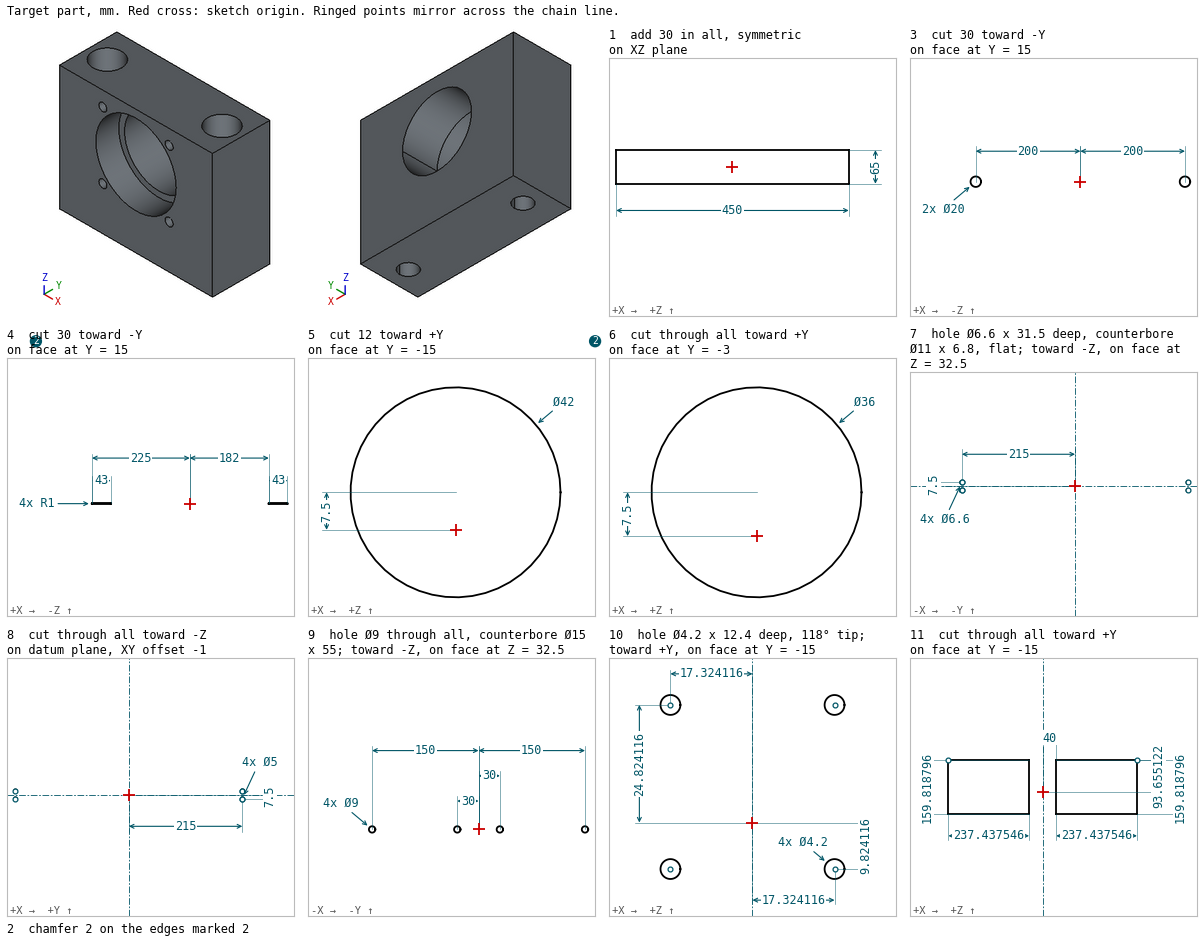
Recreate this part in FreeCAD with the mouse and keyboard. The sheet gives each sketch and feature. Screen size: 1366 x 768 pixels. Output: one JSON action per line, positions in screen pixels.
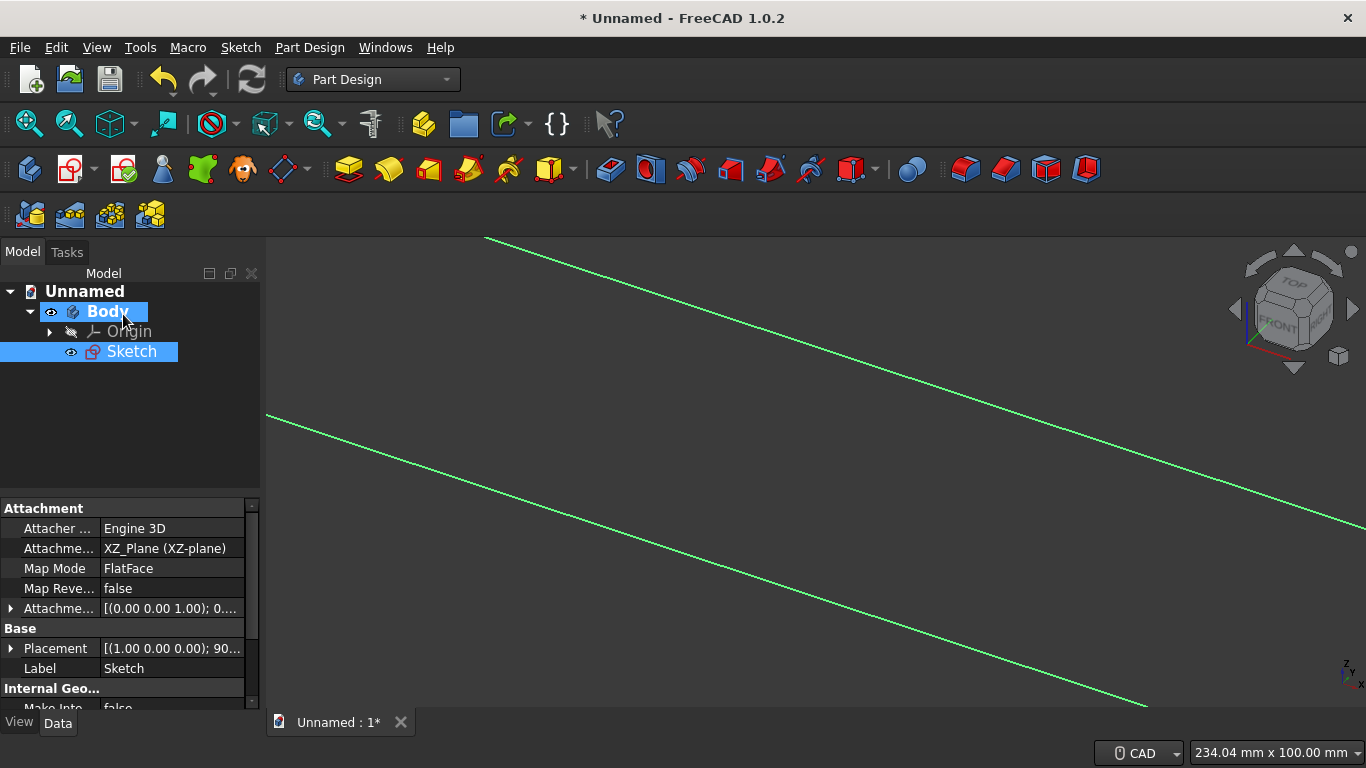
{"action": "left_click", "coordinate": [350, 170]}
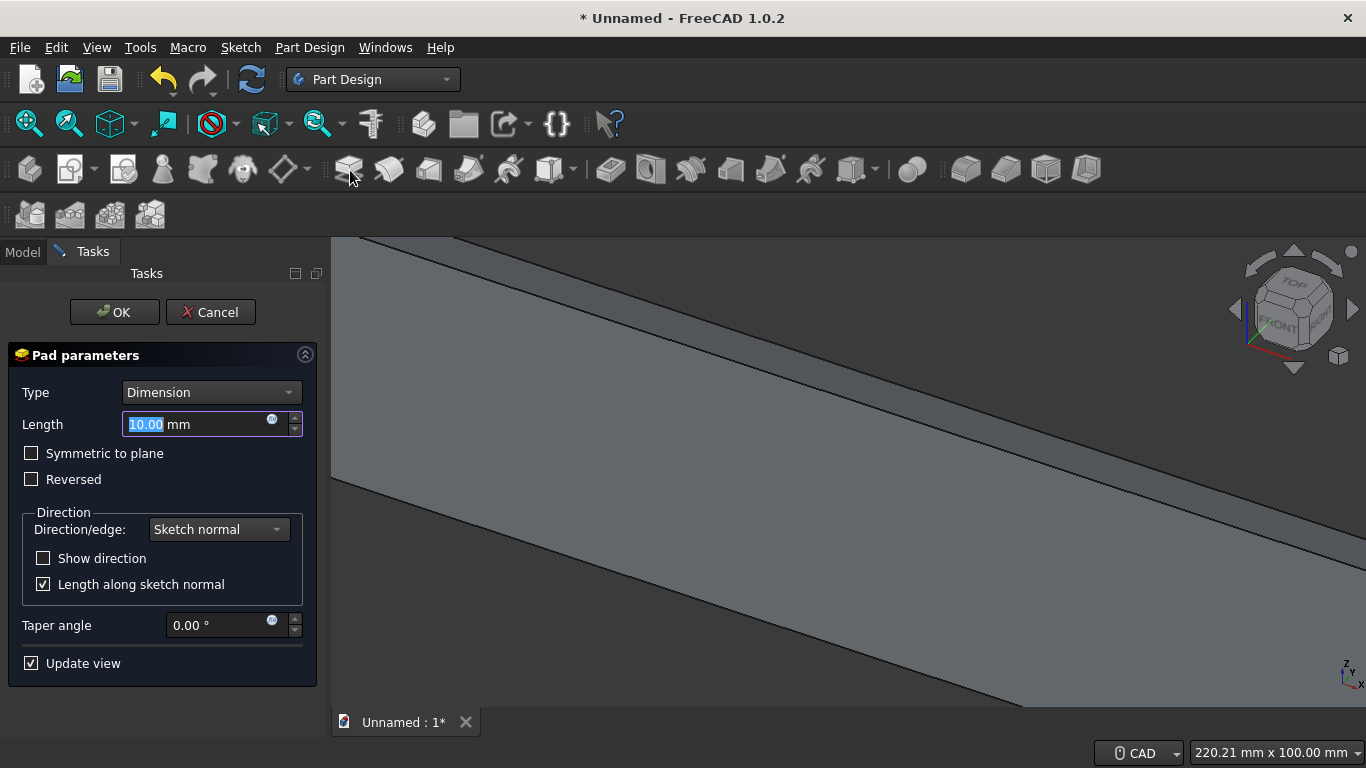
{"action": "type", "text": "30"}
{"action": "key", "text": "Tab"}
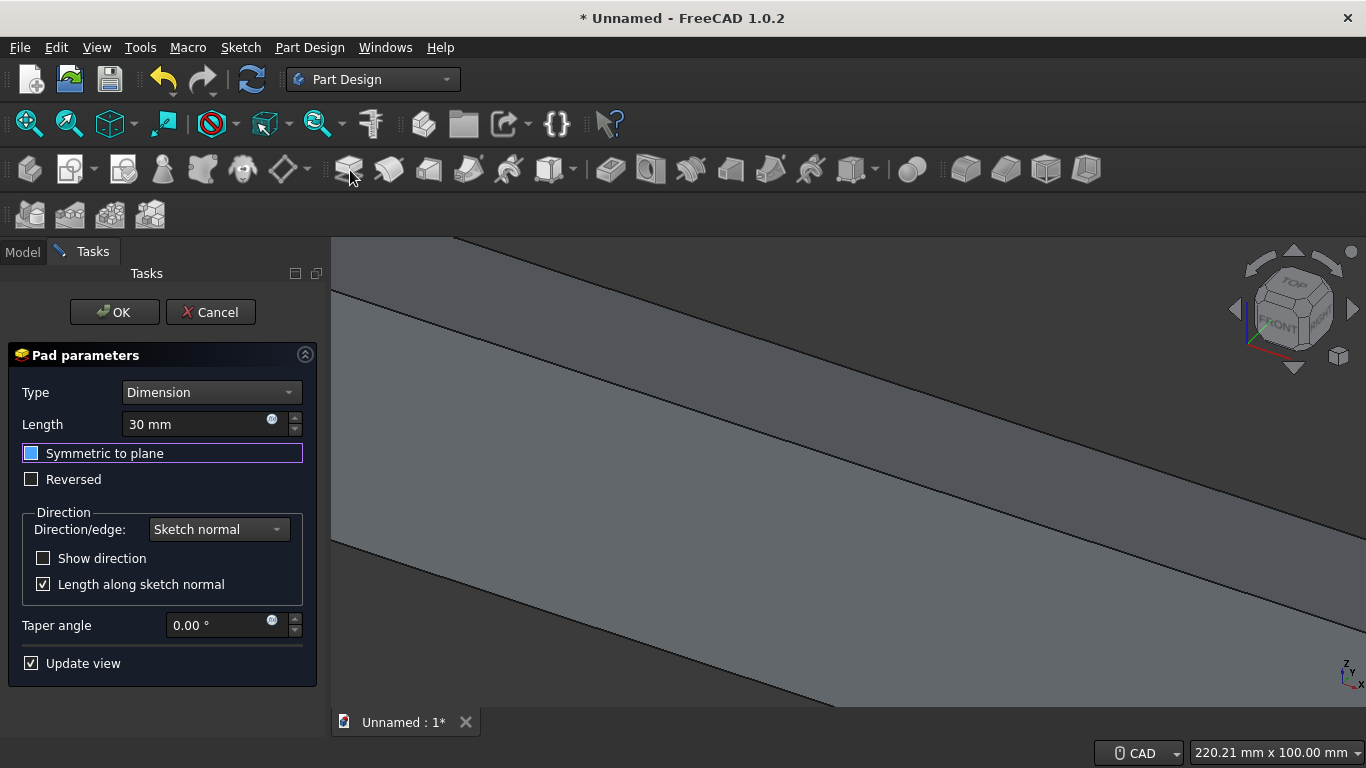
{"action": "left_click", "coordinate": [30, 453]}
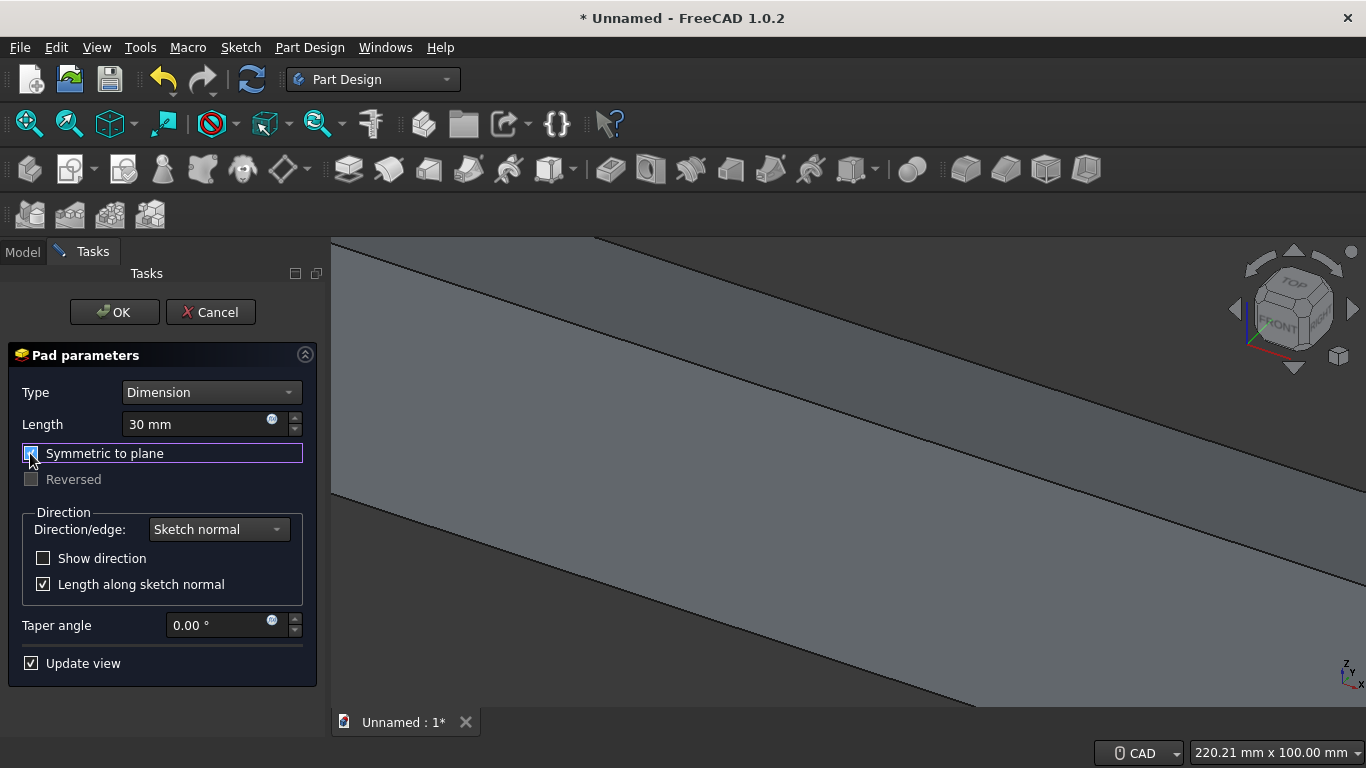
{"action": "left_click", "coordinate": [115, 312]}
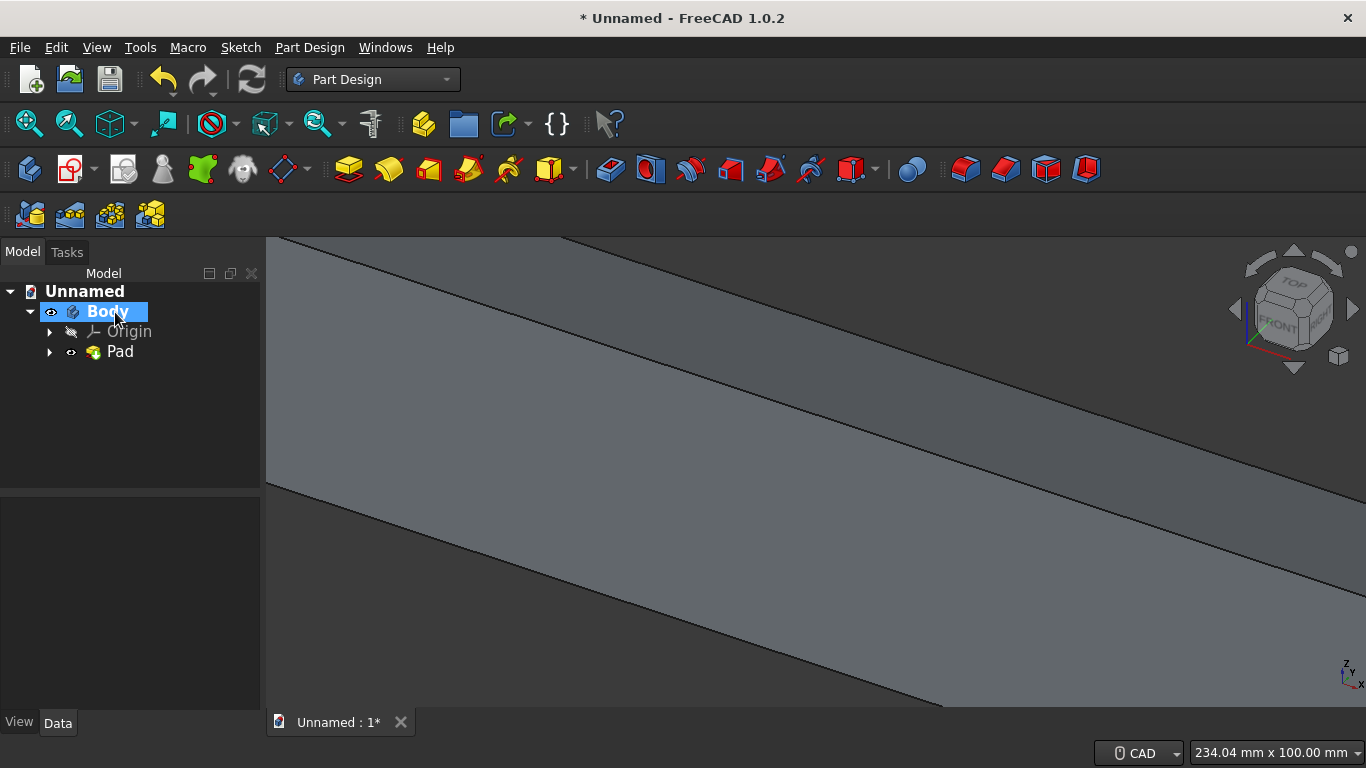
{"action": "left_click", "coordinate": [30, 124]}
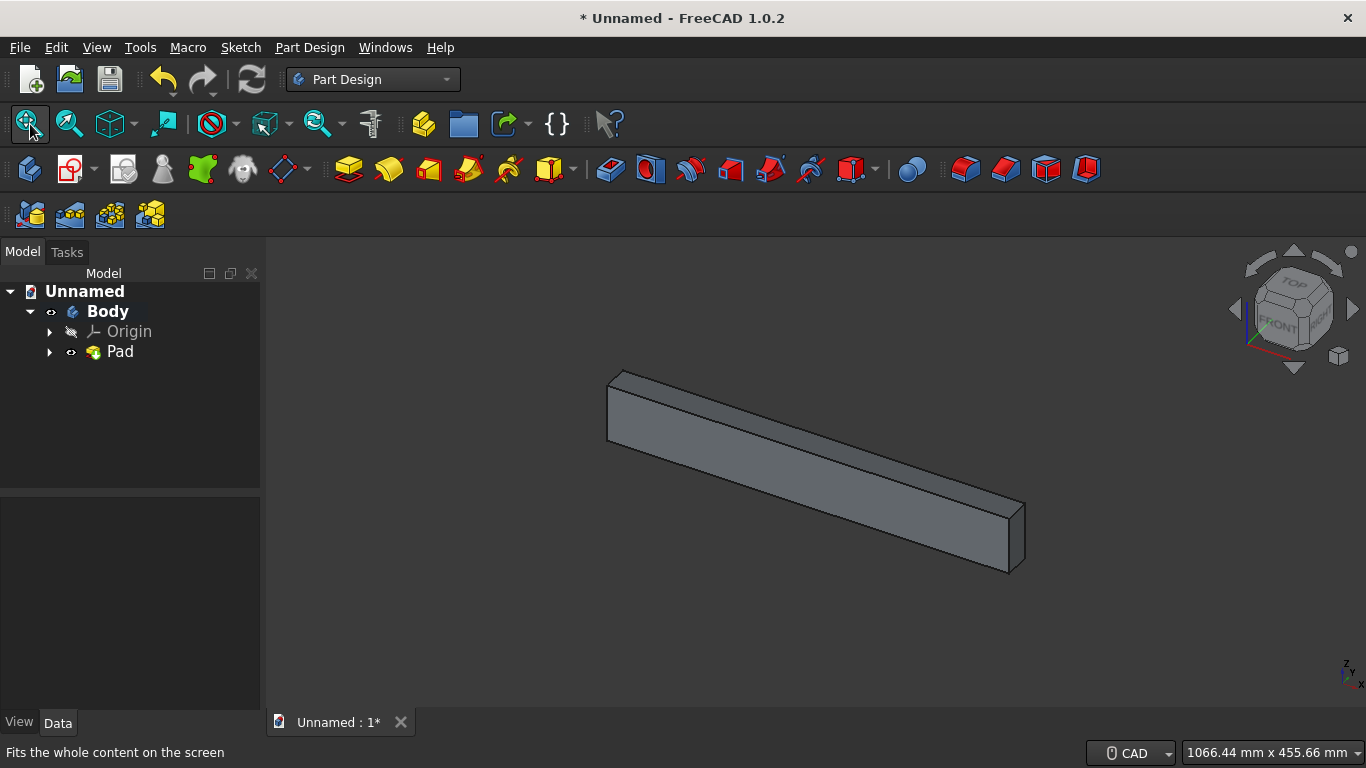
{"action": "left_click", "coordinate": [1017, 510]}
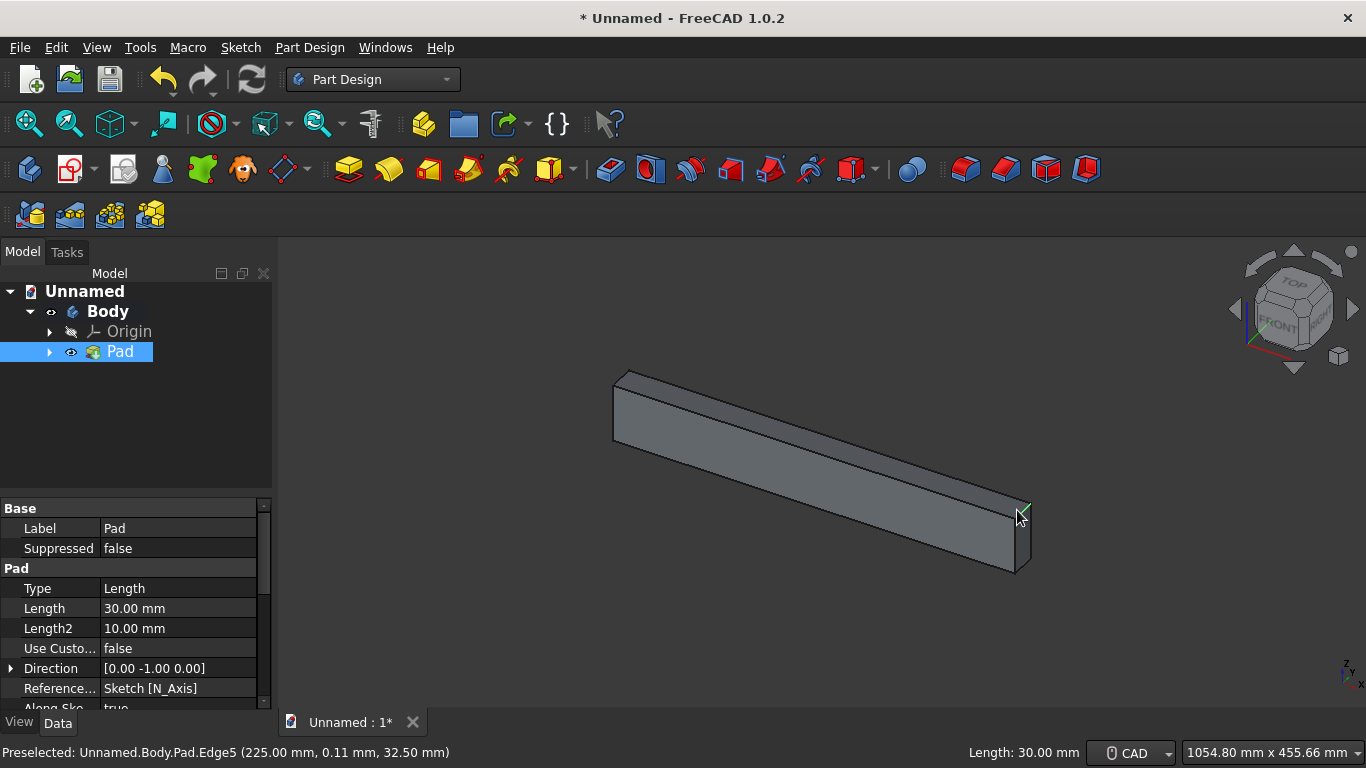
{"action": "key", "text": "0"}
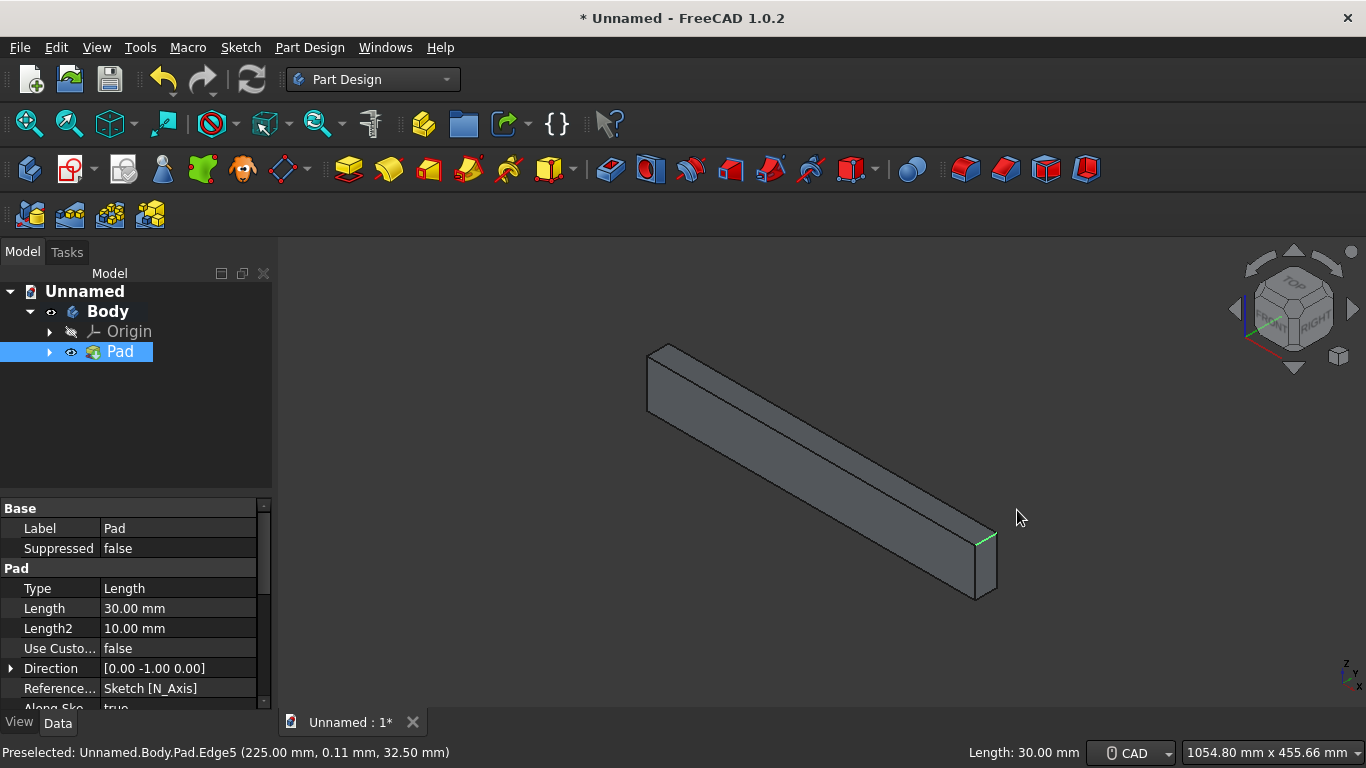
{"action": "key", "text": "2"}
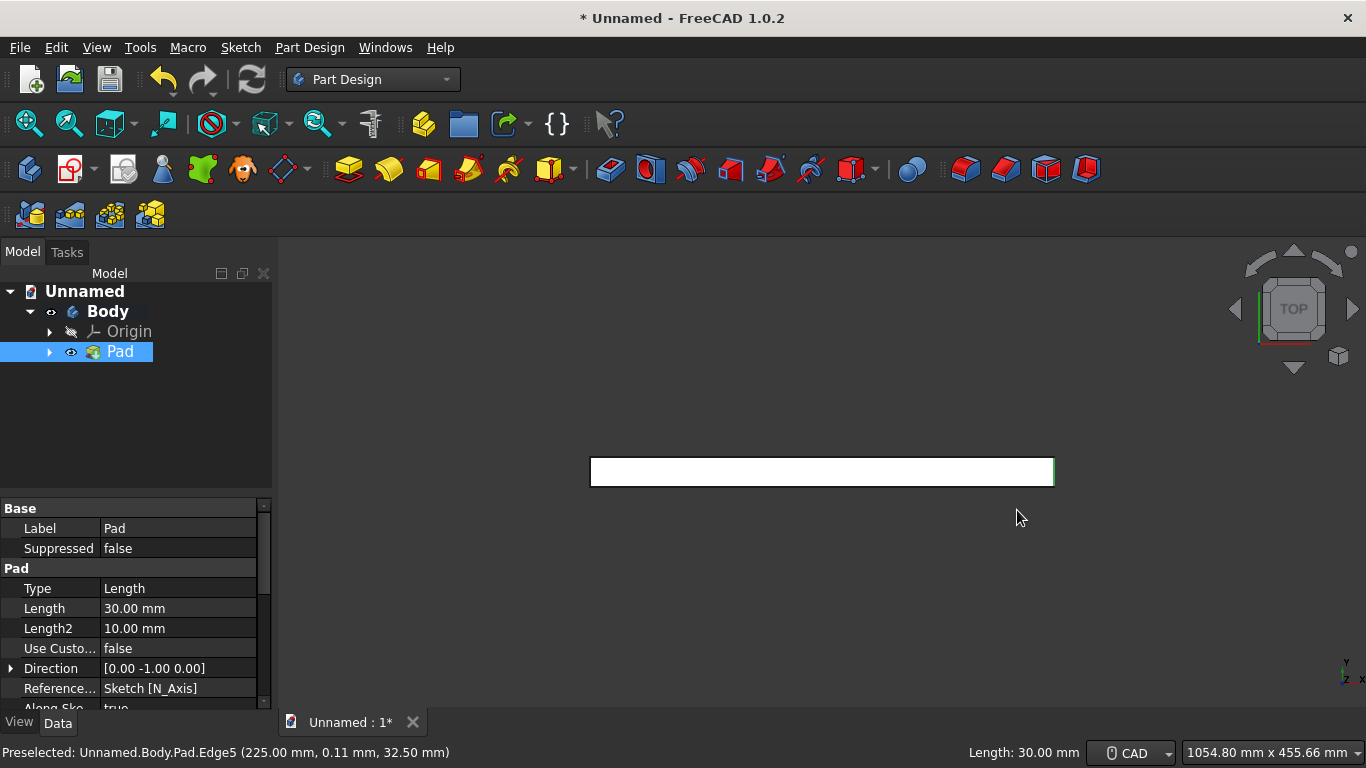
{"action": "key", "text": "v f"}